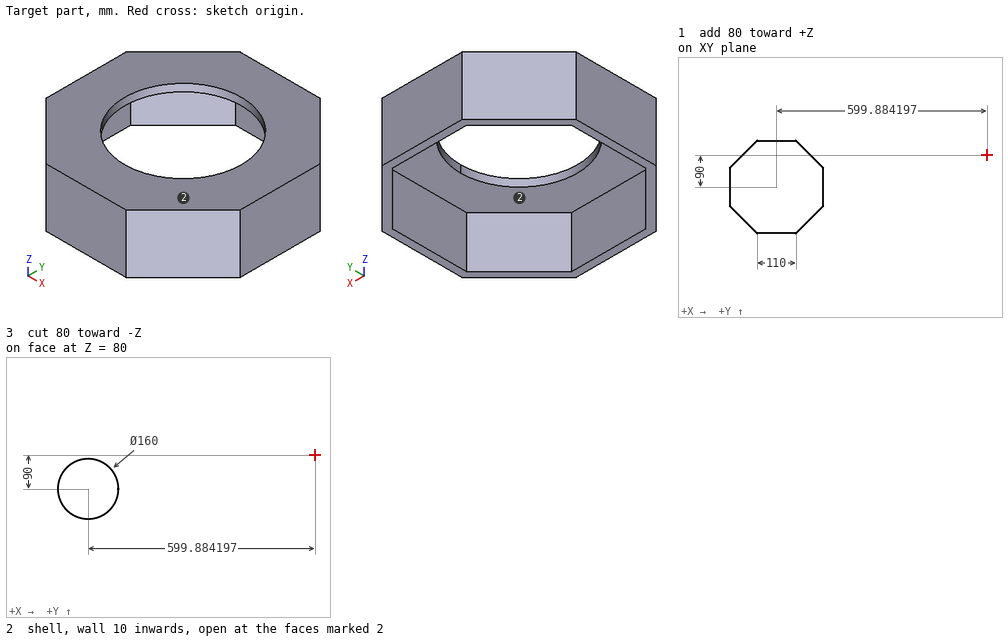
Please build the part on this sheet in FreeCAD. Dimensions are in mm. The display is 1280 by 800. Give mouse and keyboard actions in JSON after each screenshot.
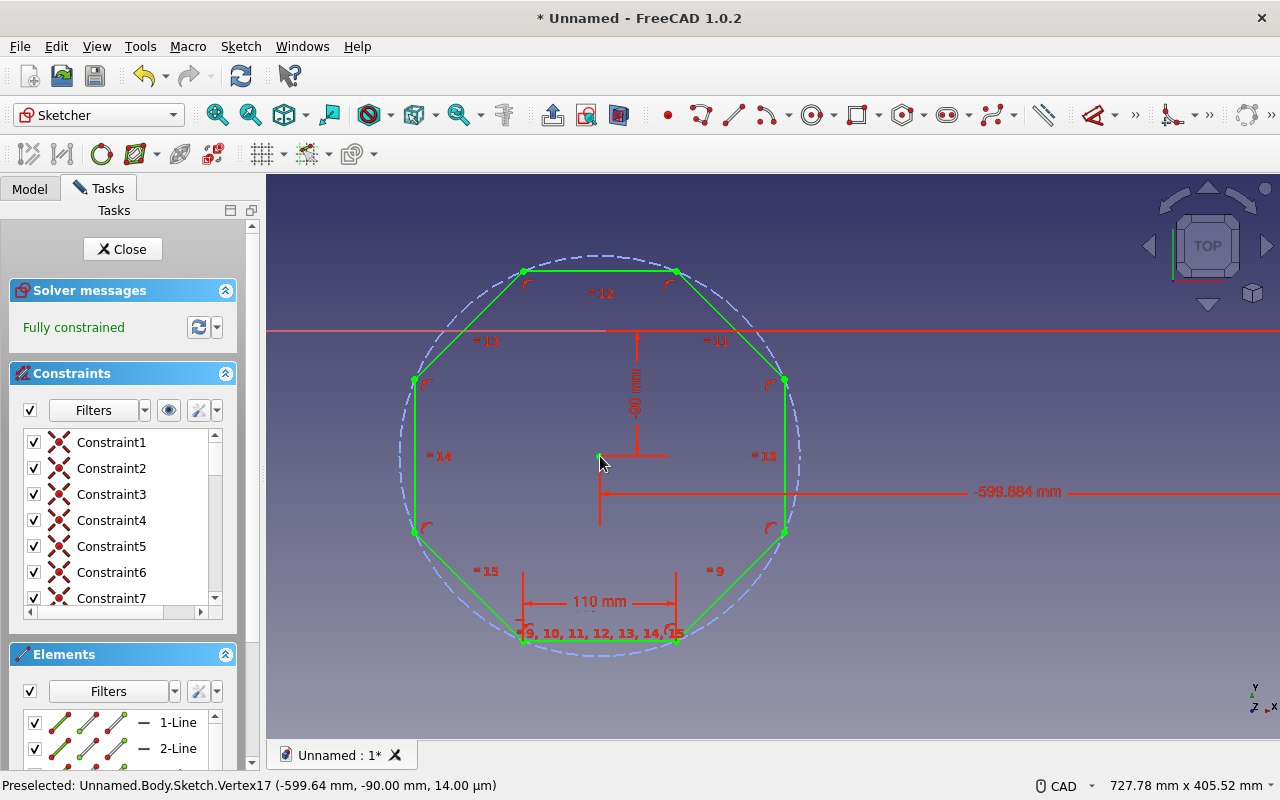
{"action": "left_click", "coordinate": [123, 249]}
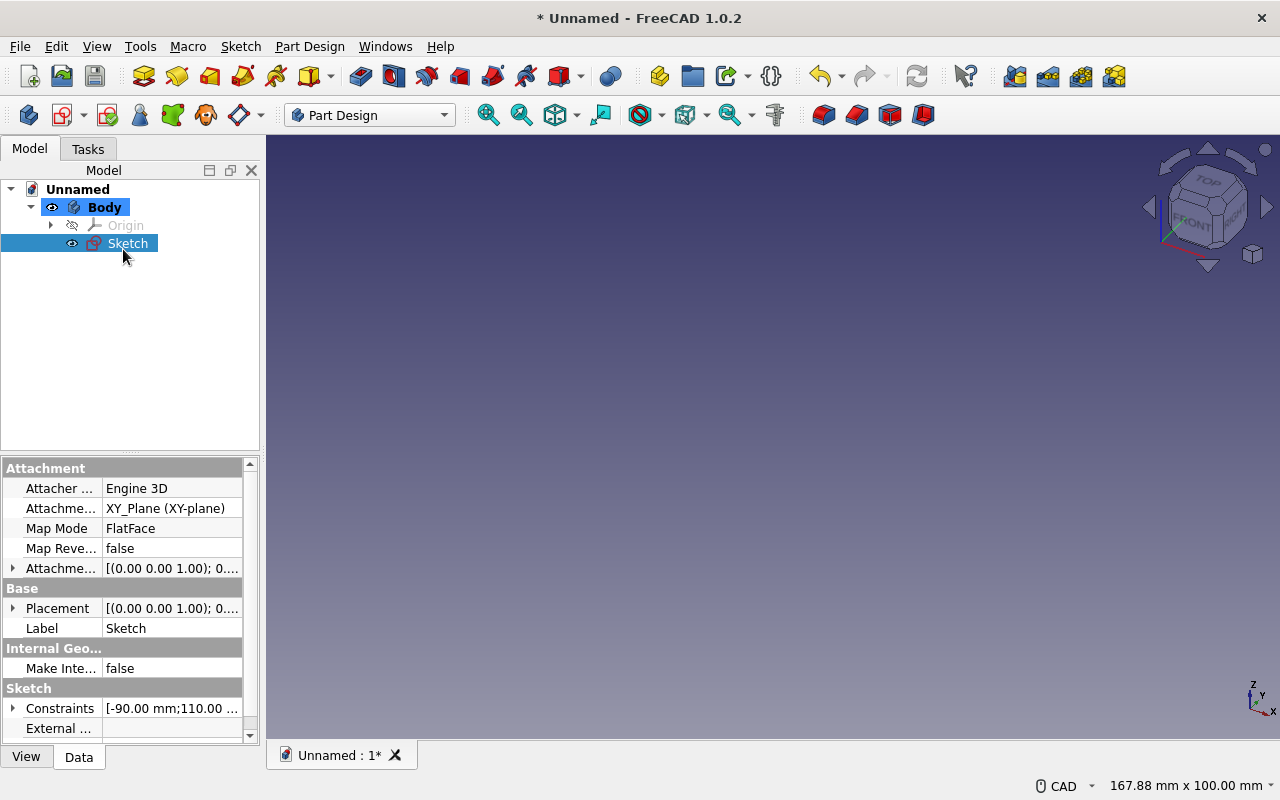
{"action": "left_click", "coordinate": [144, 76]}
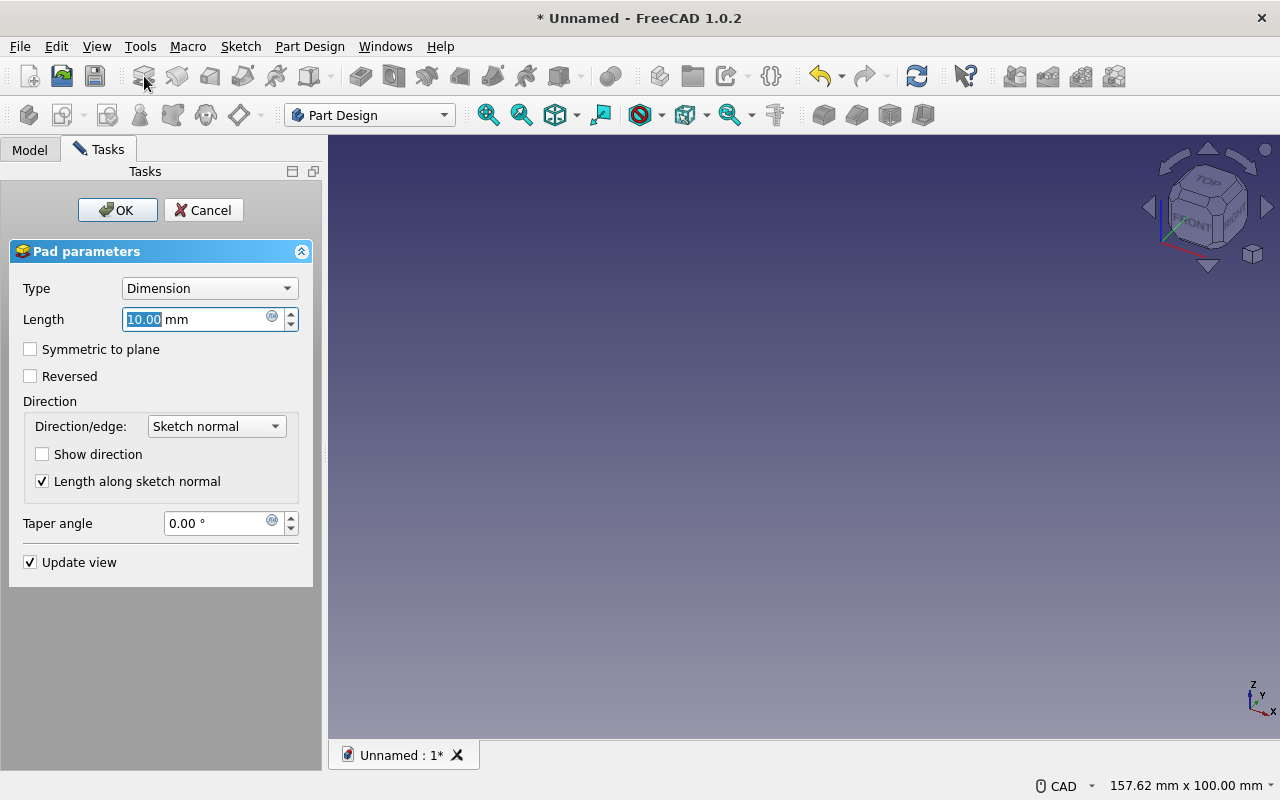
{"action": "type", "text": "80"}
{"action": "key", "text": "Tab"}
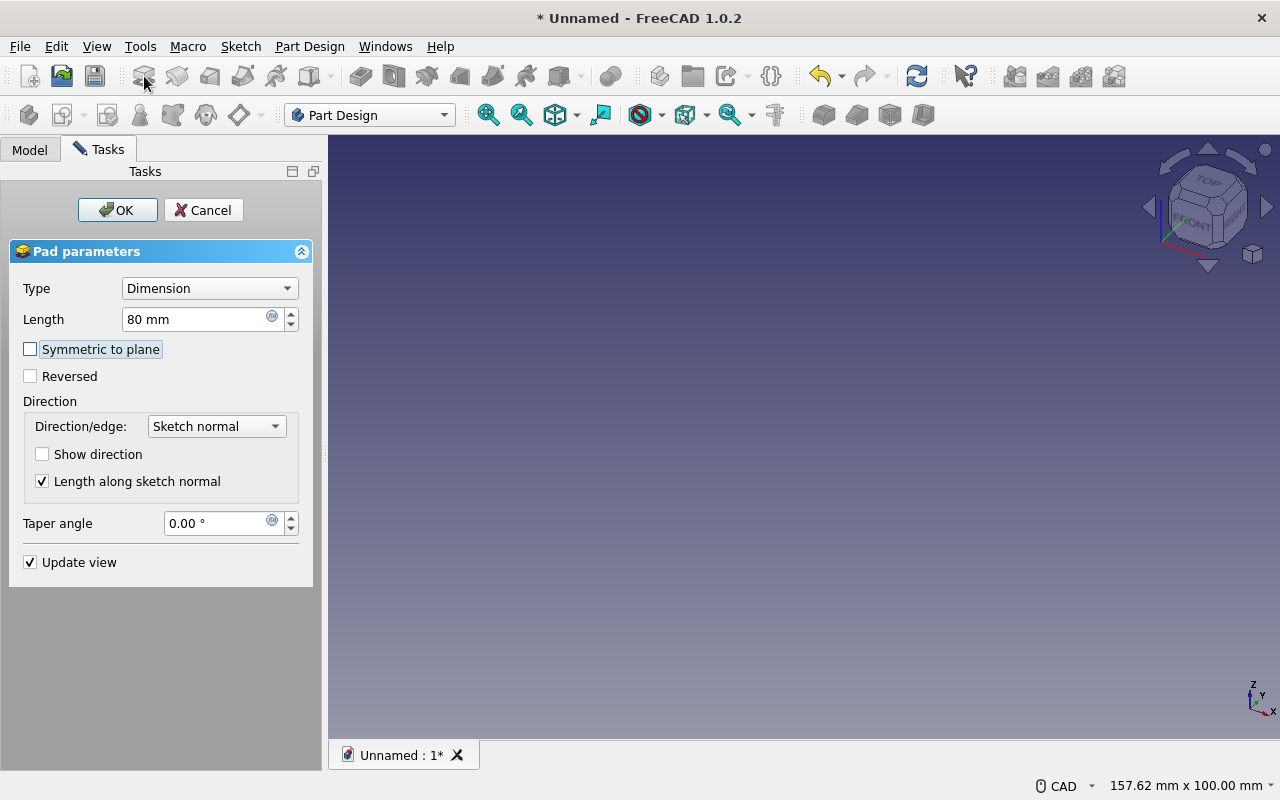
{"action": "left_click", "coordinate": [118, 210]}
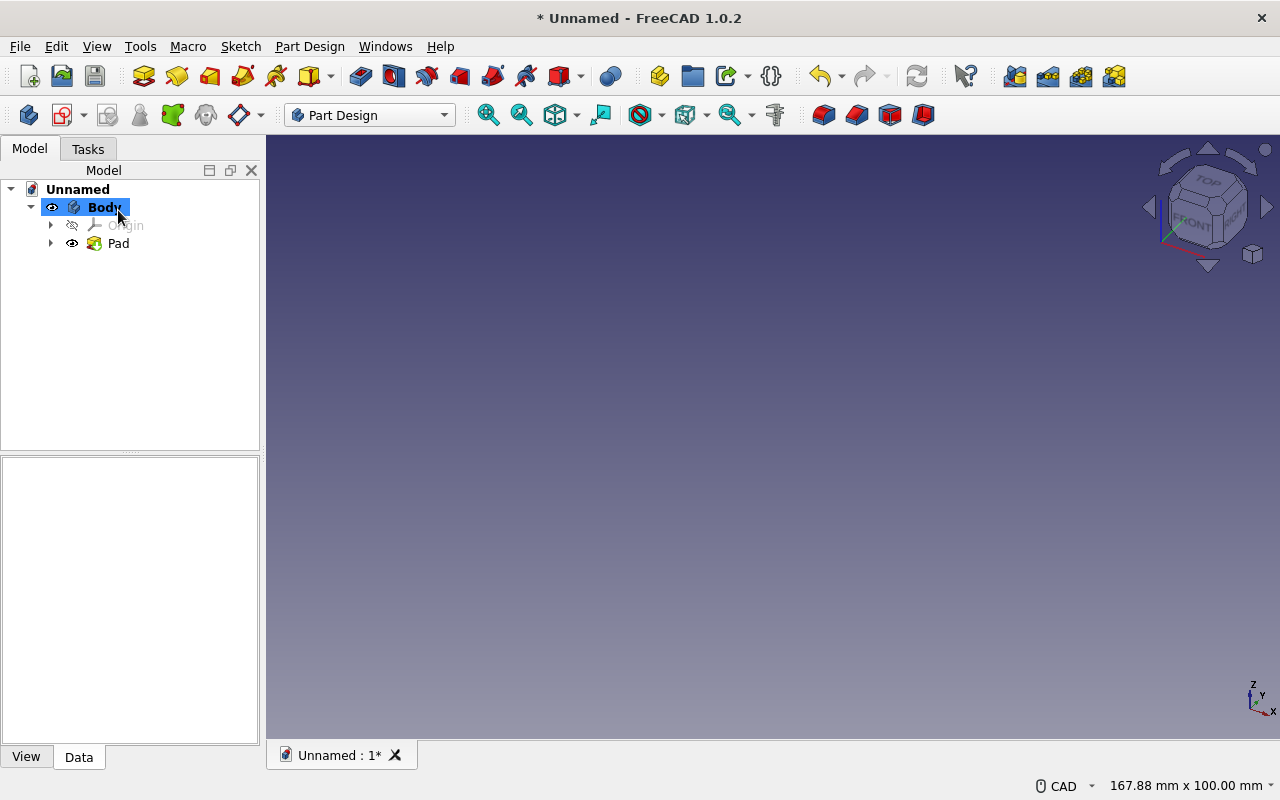
{"action": "key", "text": "v f"}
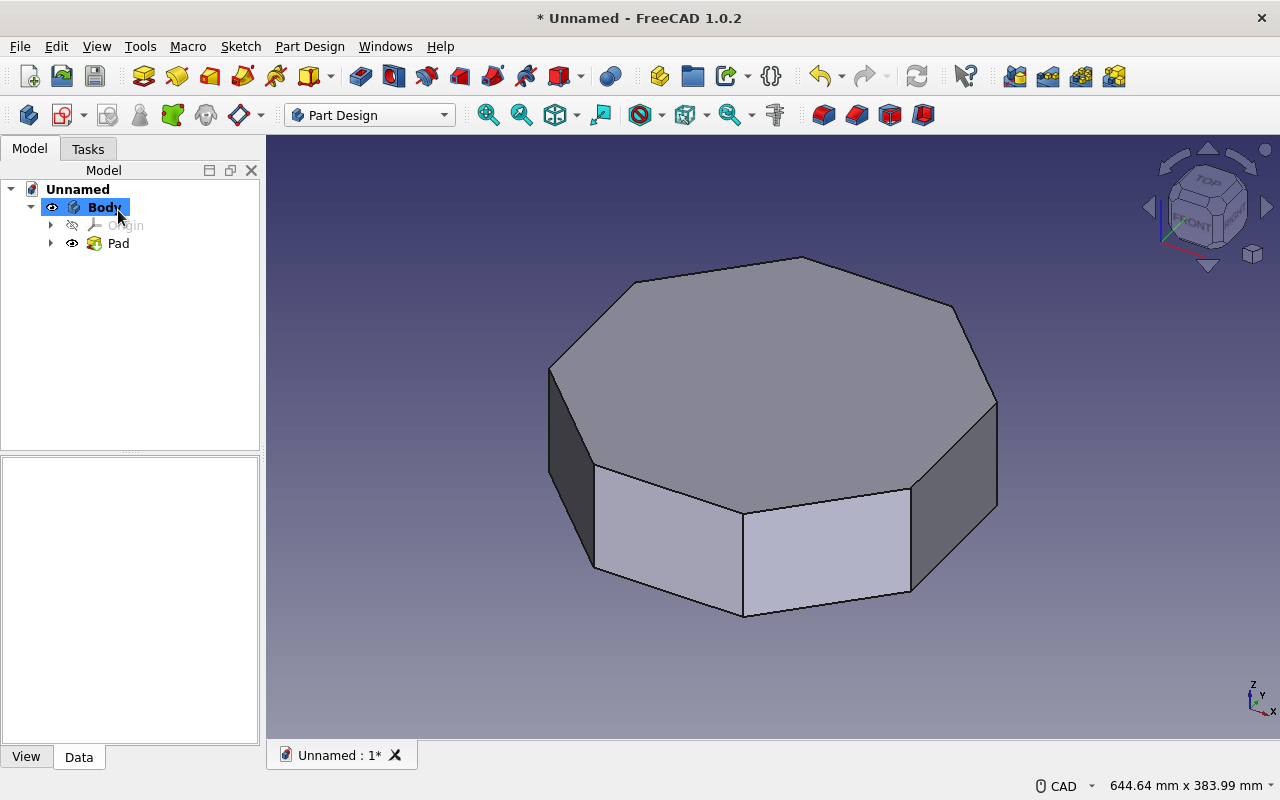
{"action": "key", "text": "0"}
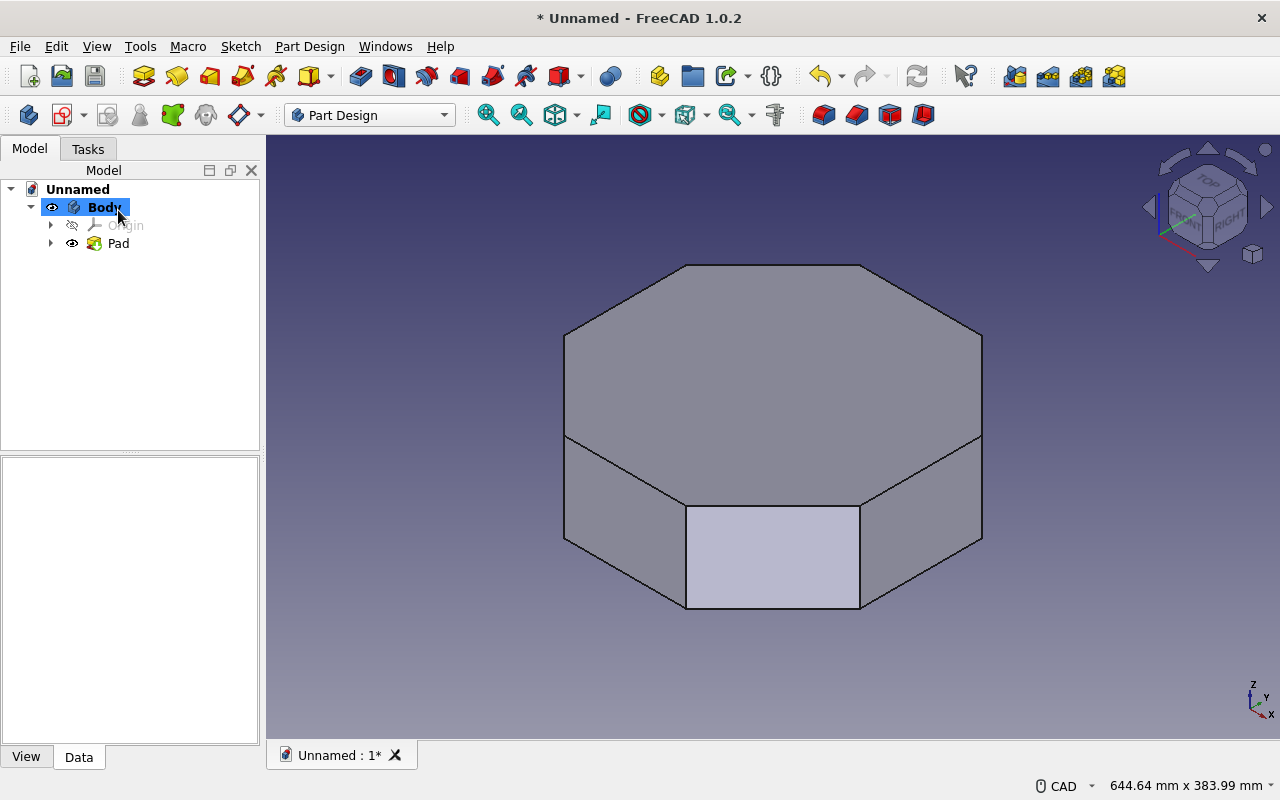
{"action": "key", "text": "2"}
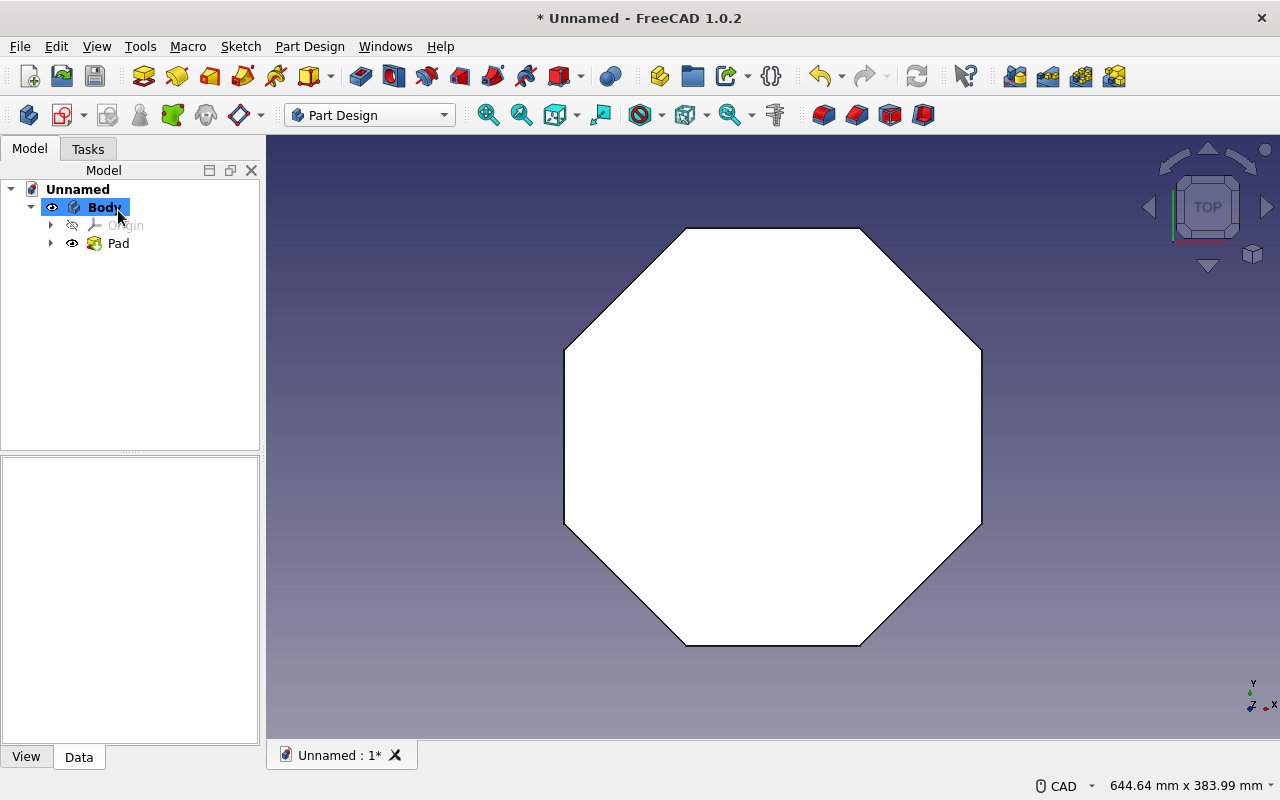
{"action": "key", "text": "1"}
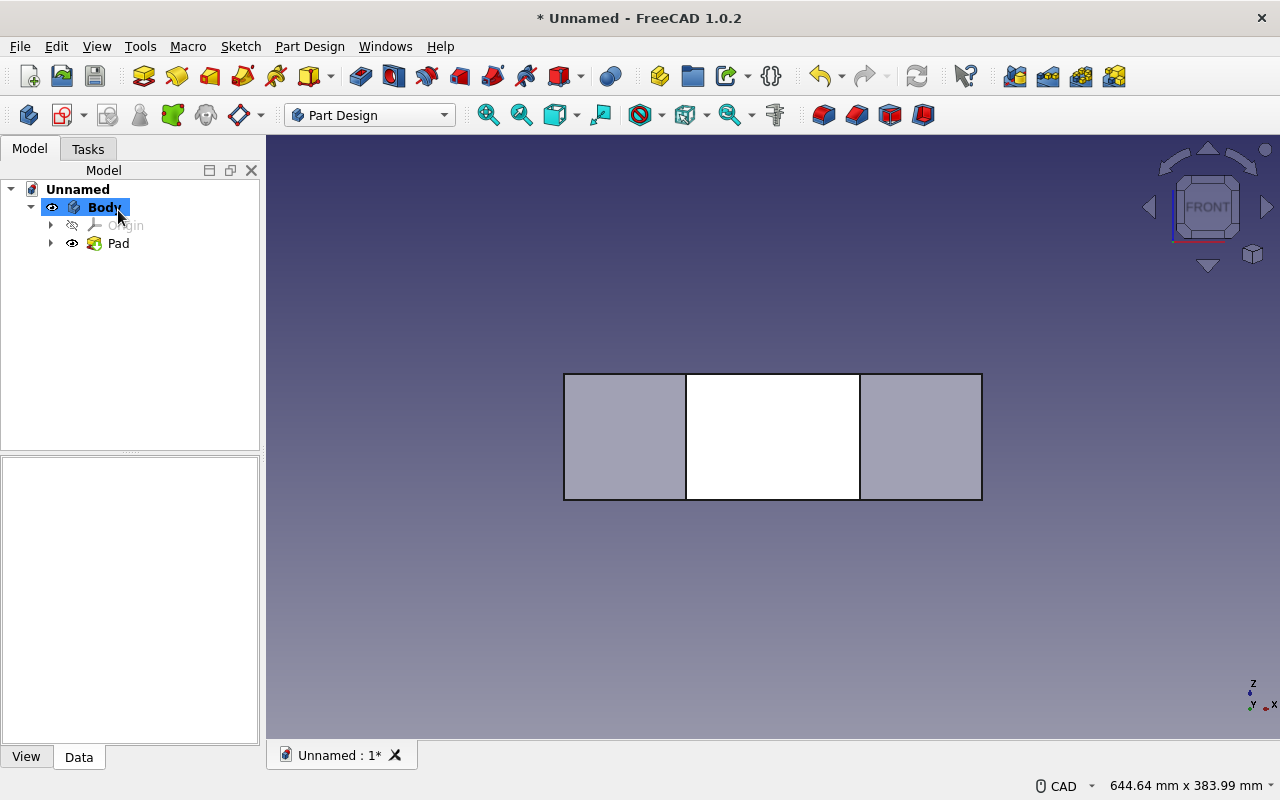
{"action": "key", "text": "v f"}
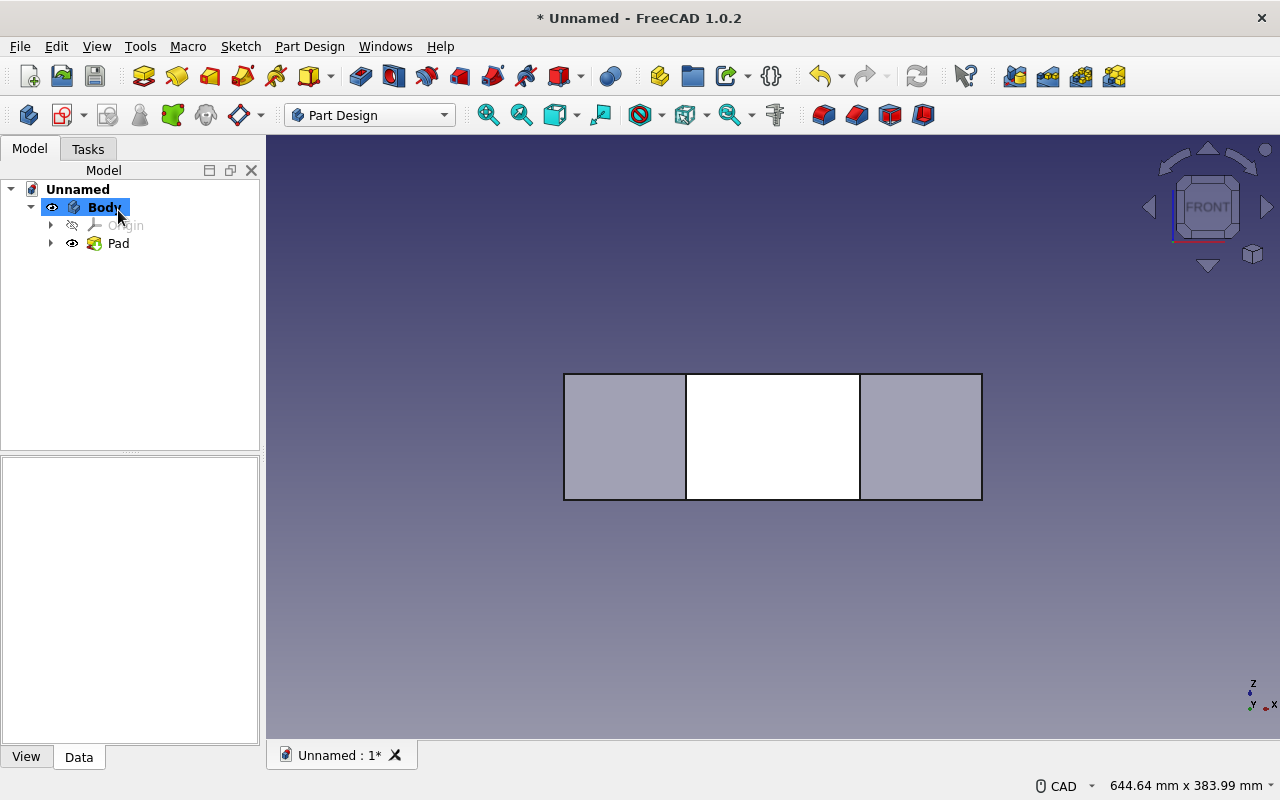
{"action": "key", "text": "3"}